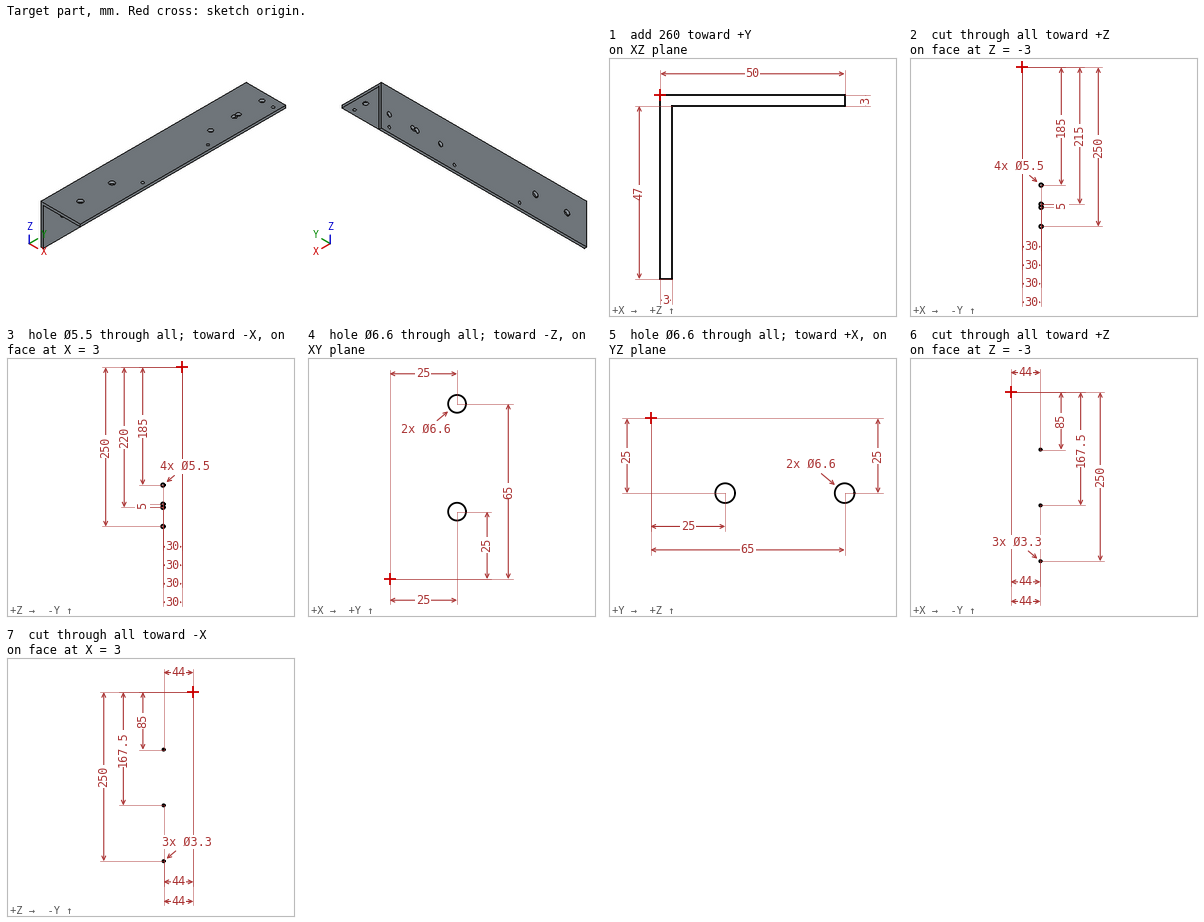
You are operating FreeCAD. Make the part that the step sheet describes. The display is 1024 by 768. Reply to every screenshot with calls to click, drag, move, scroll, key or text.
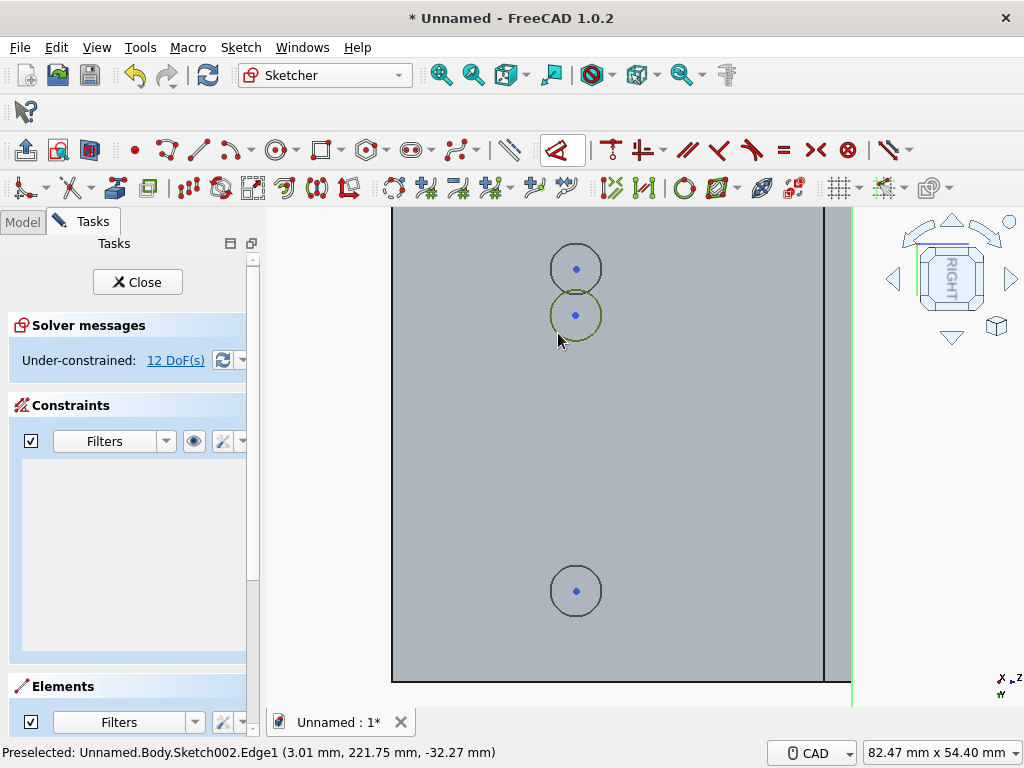
scroll(577, 592, down, 4)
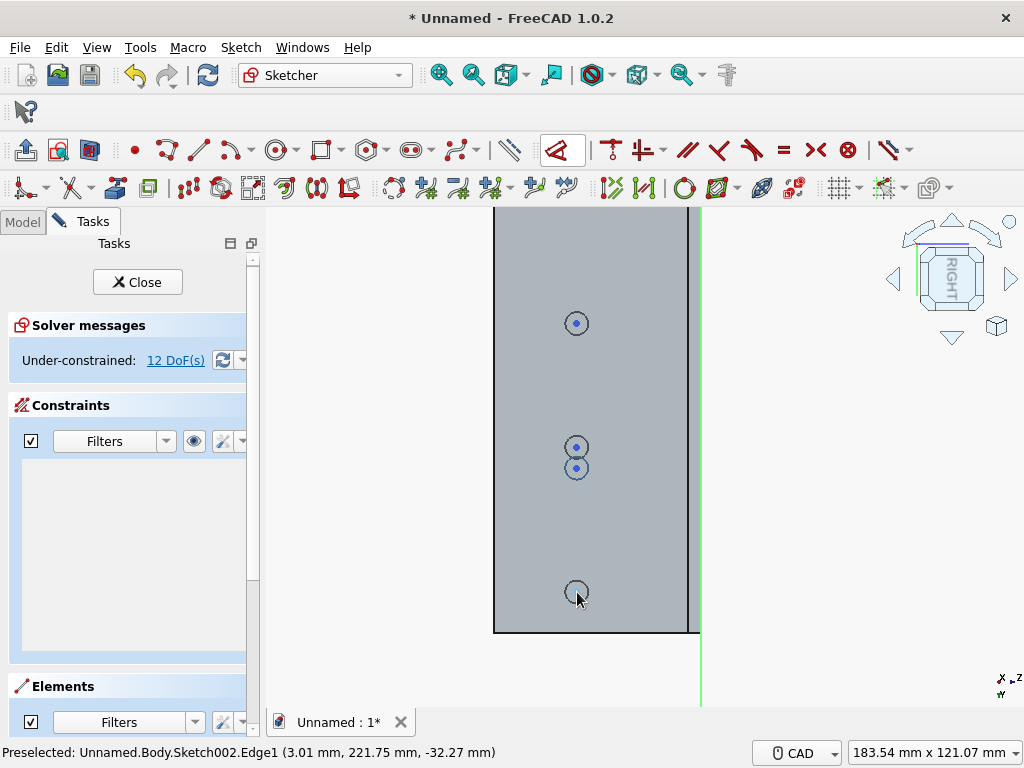
click(585, 315)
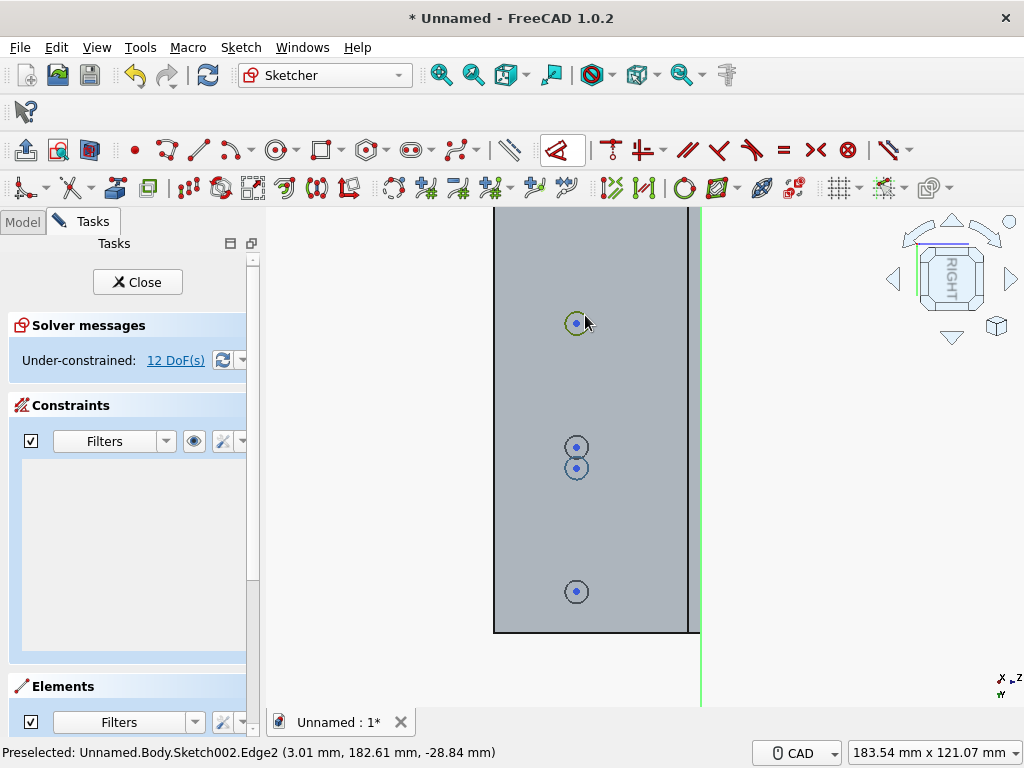
click(585, 584)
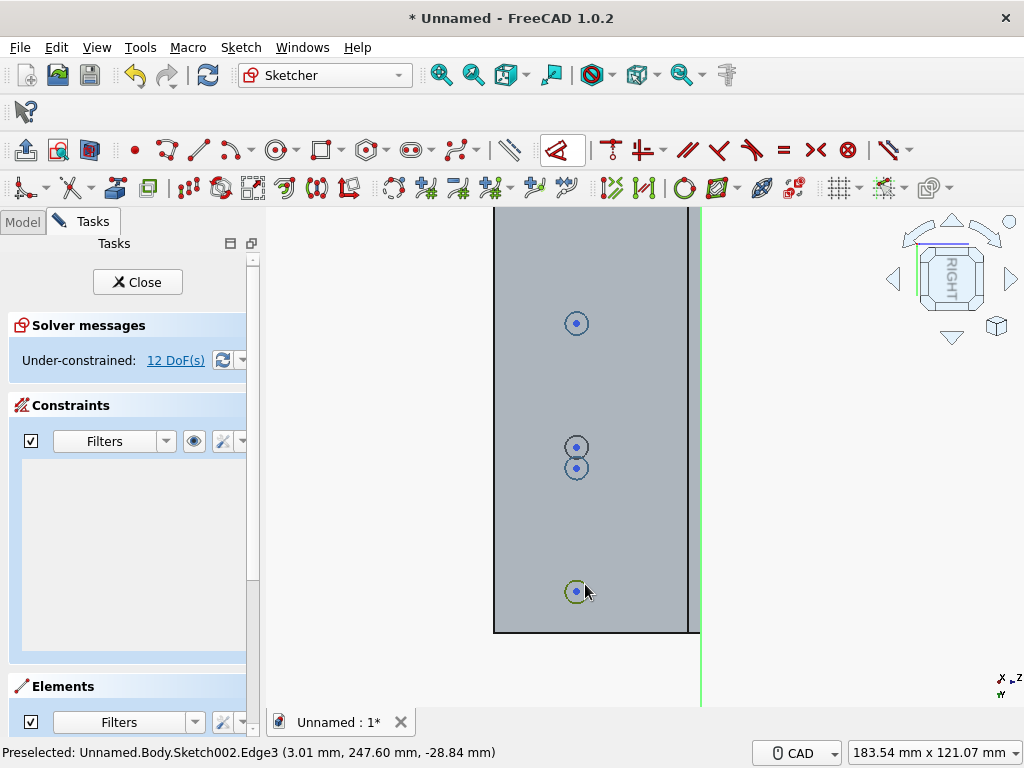
click(585, 439)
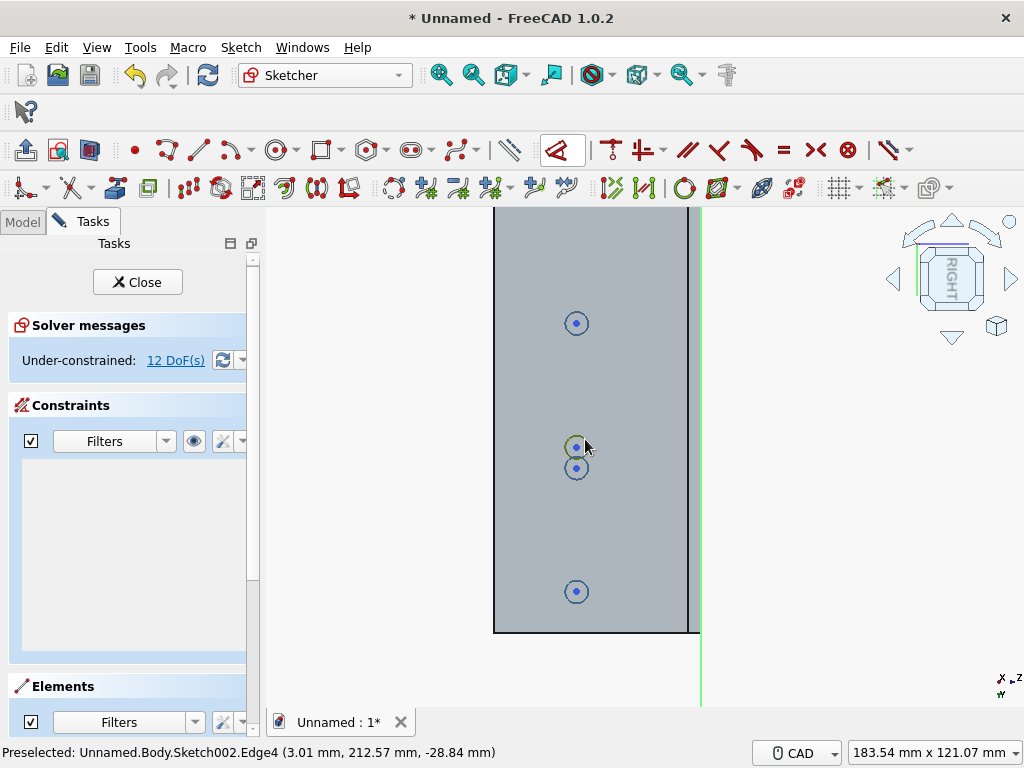
key(e)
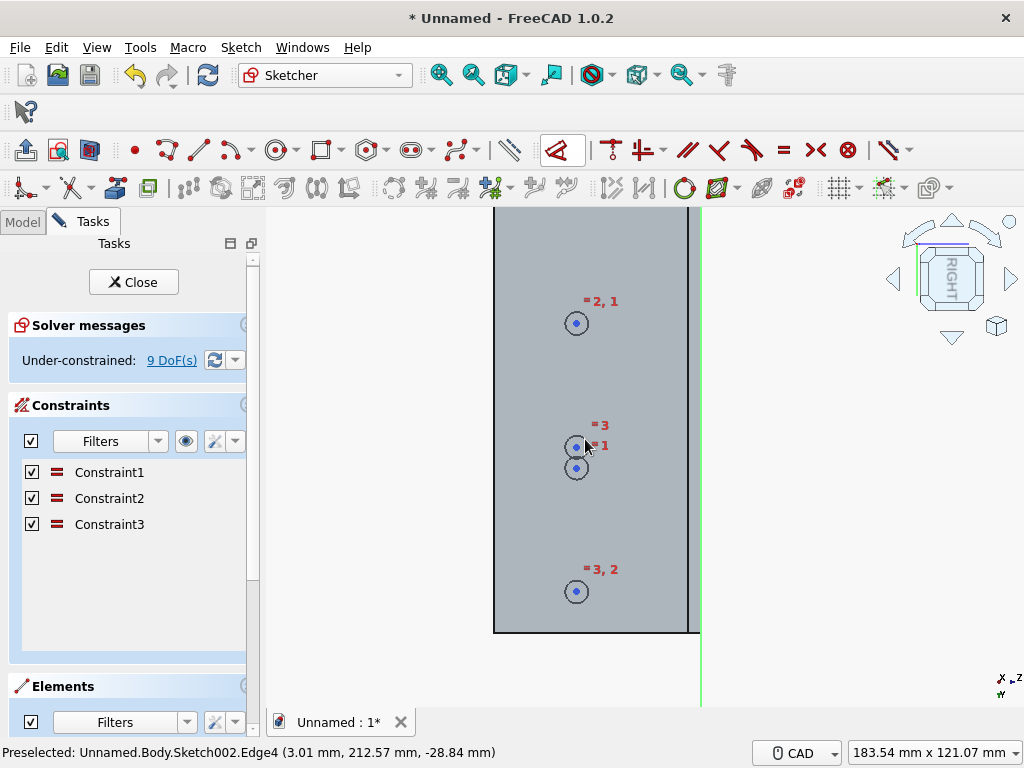
scroll(569, 476, up, 3)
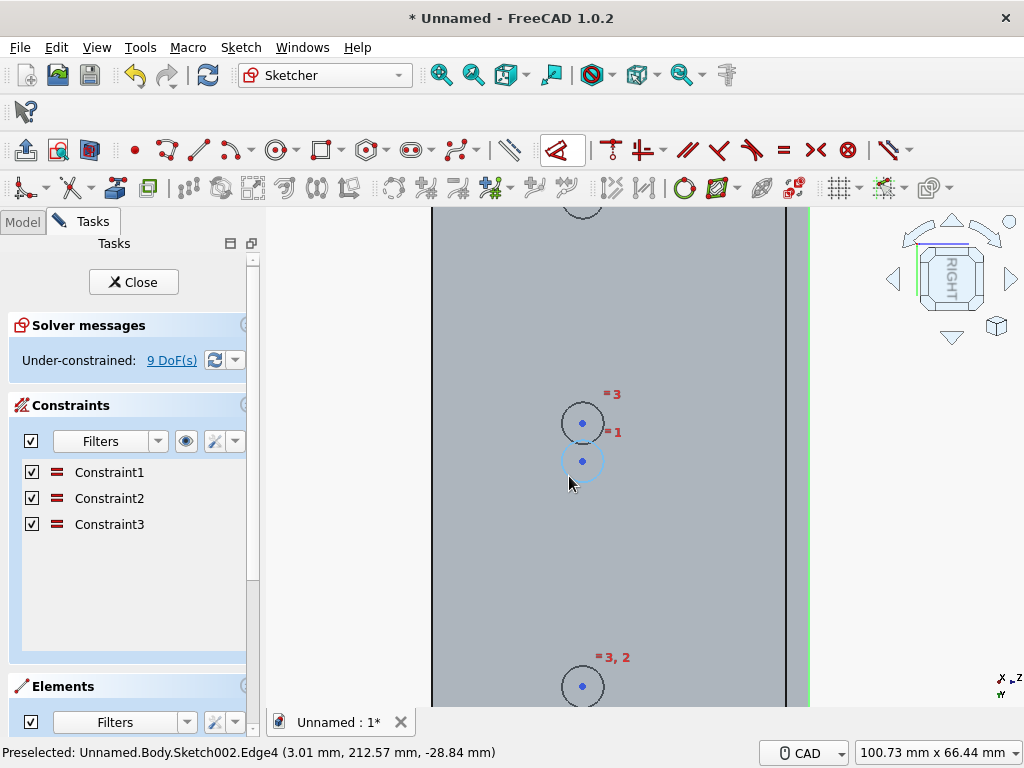
click(568, 476)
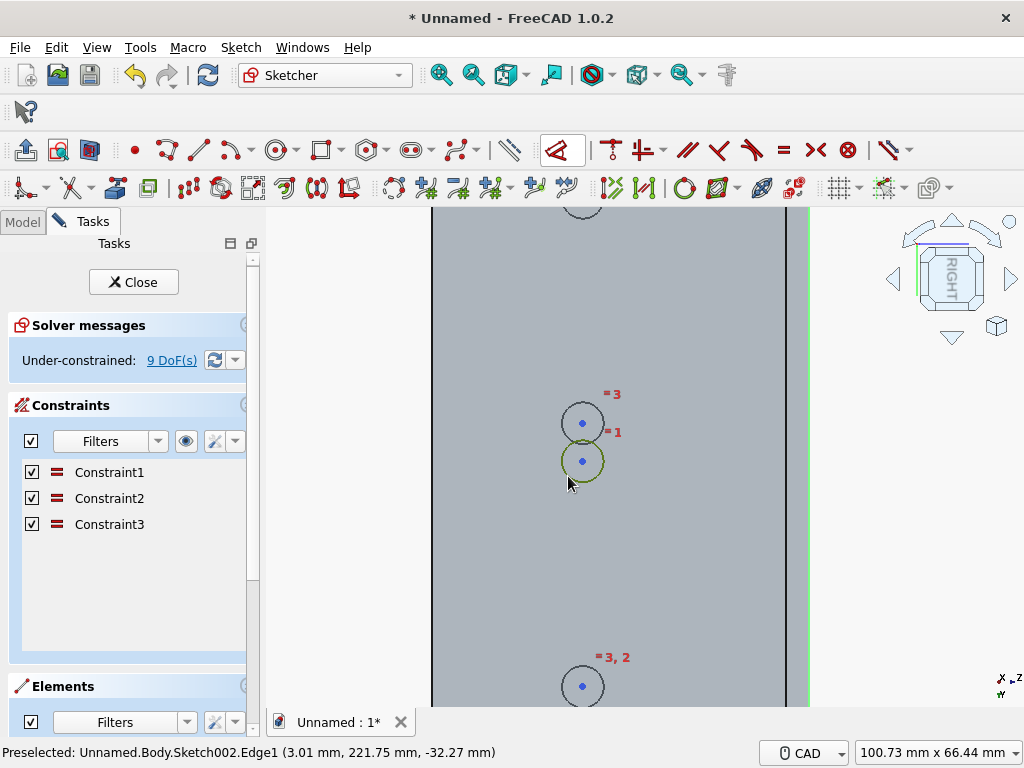
key(k)
key(o)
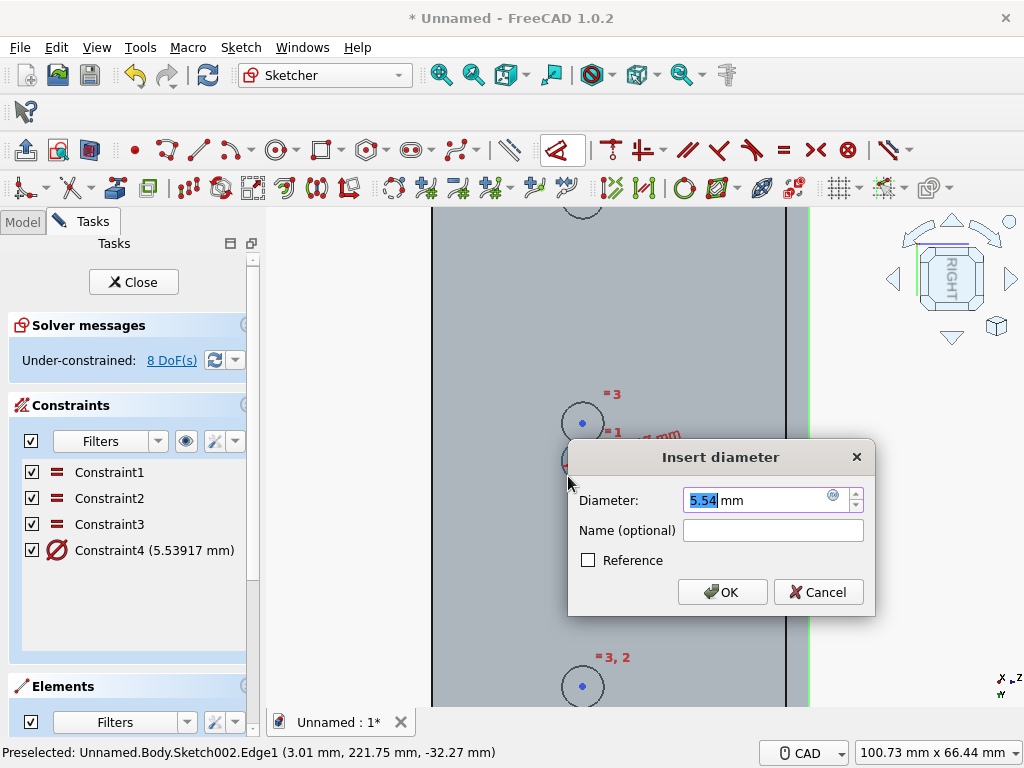
text(5.5)
key(Return)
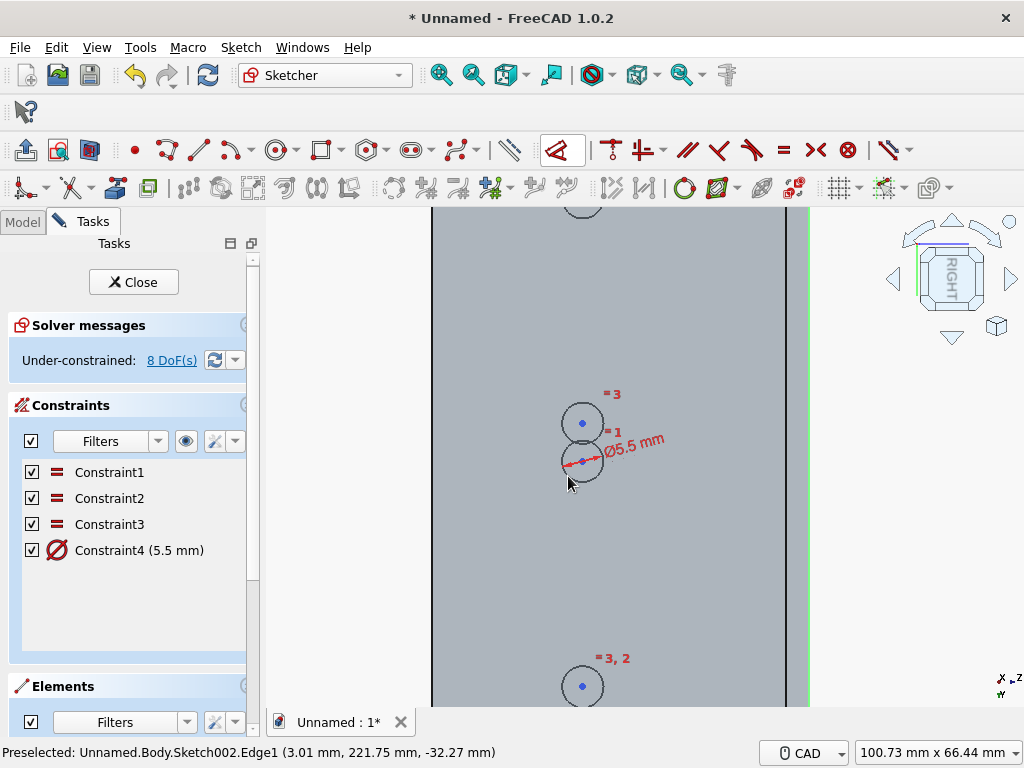
click(583, 461)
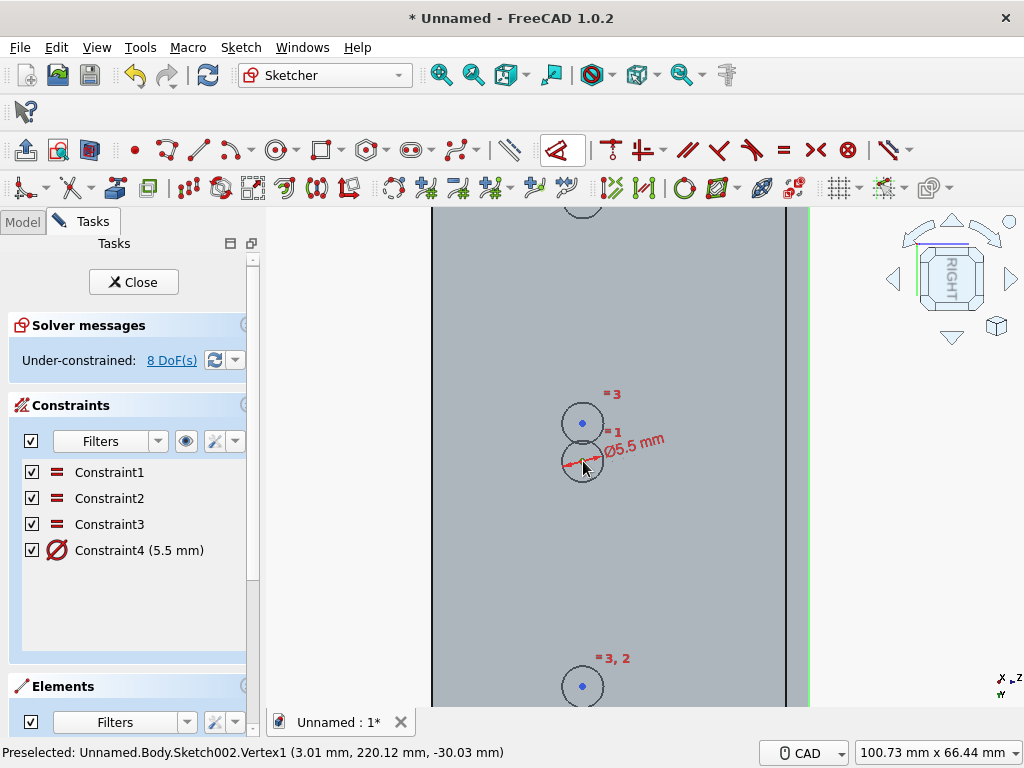
key(l)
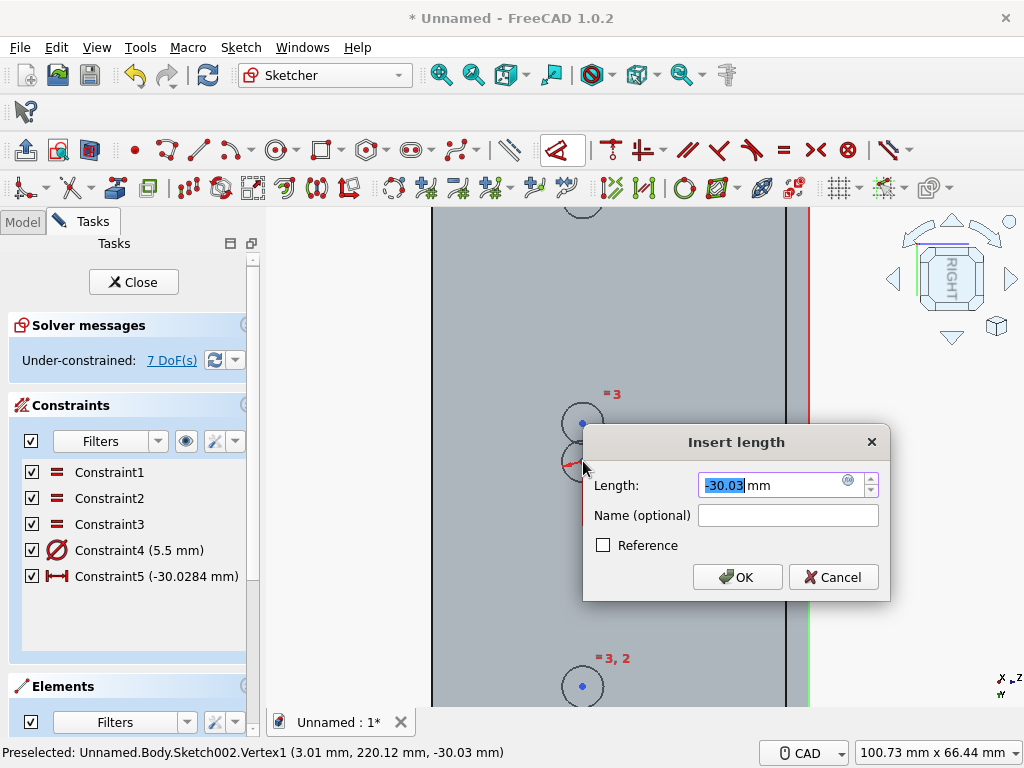
text(-30)
key(Return)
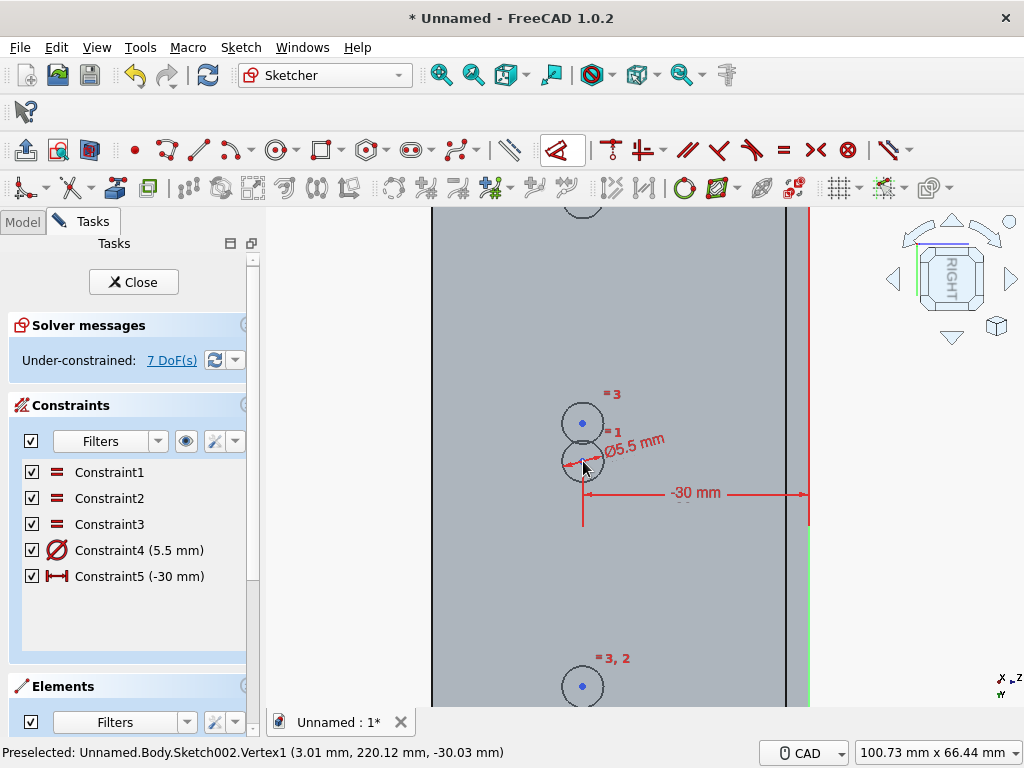
scroll(569, 476, down, 3)